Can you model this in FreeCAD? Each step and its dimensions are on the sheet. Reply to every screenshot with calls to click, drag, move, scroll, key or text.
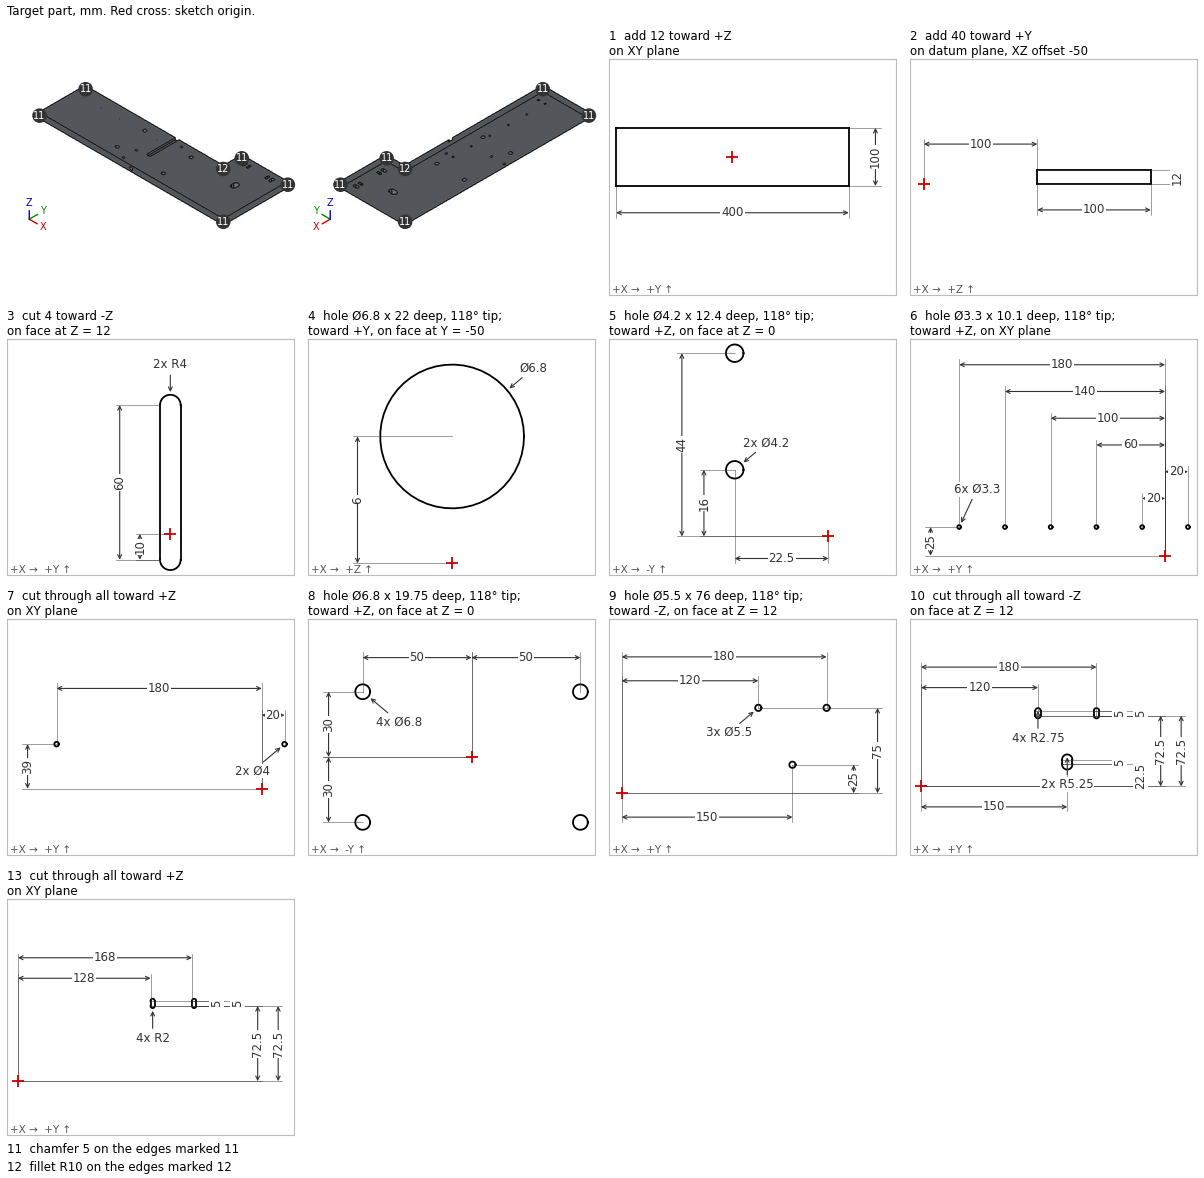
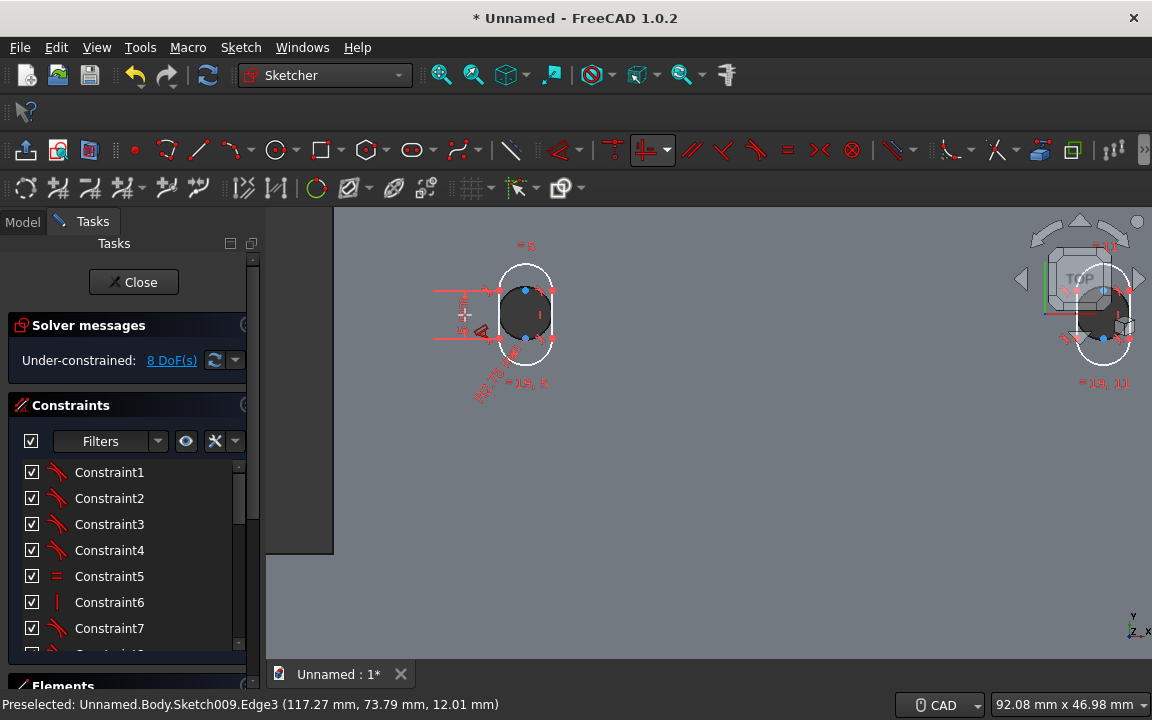
scroll(499, 325, down, 4)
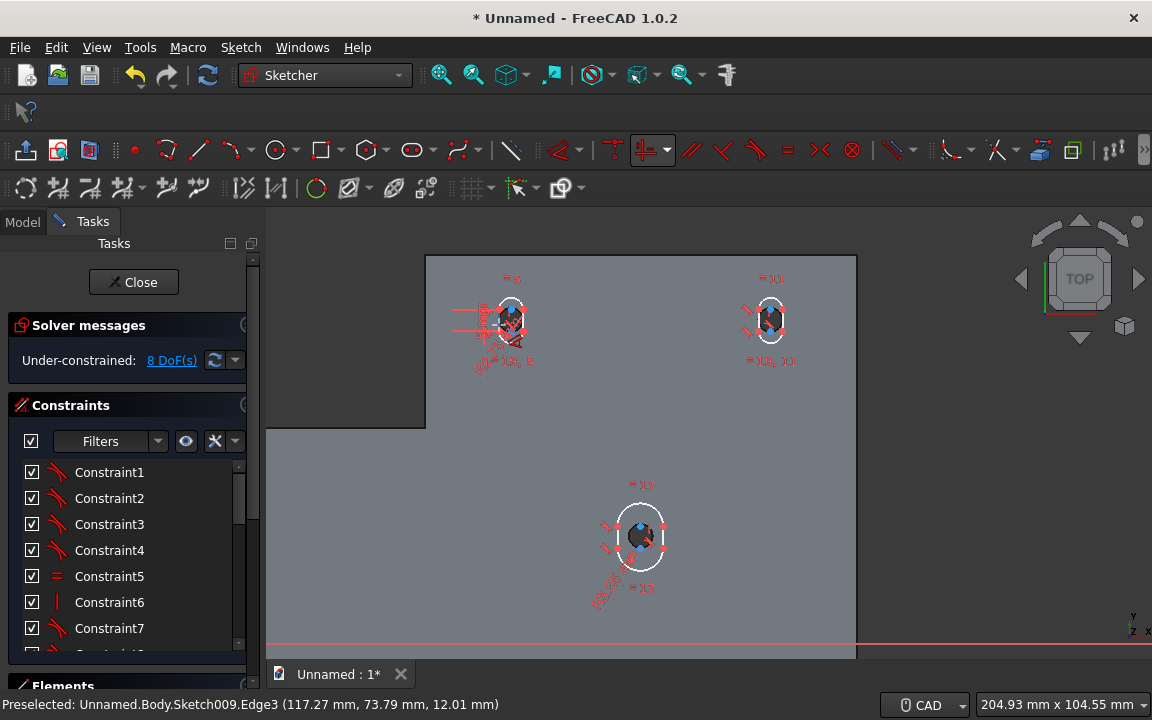
scroll(759, 325, up, 4)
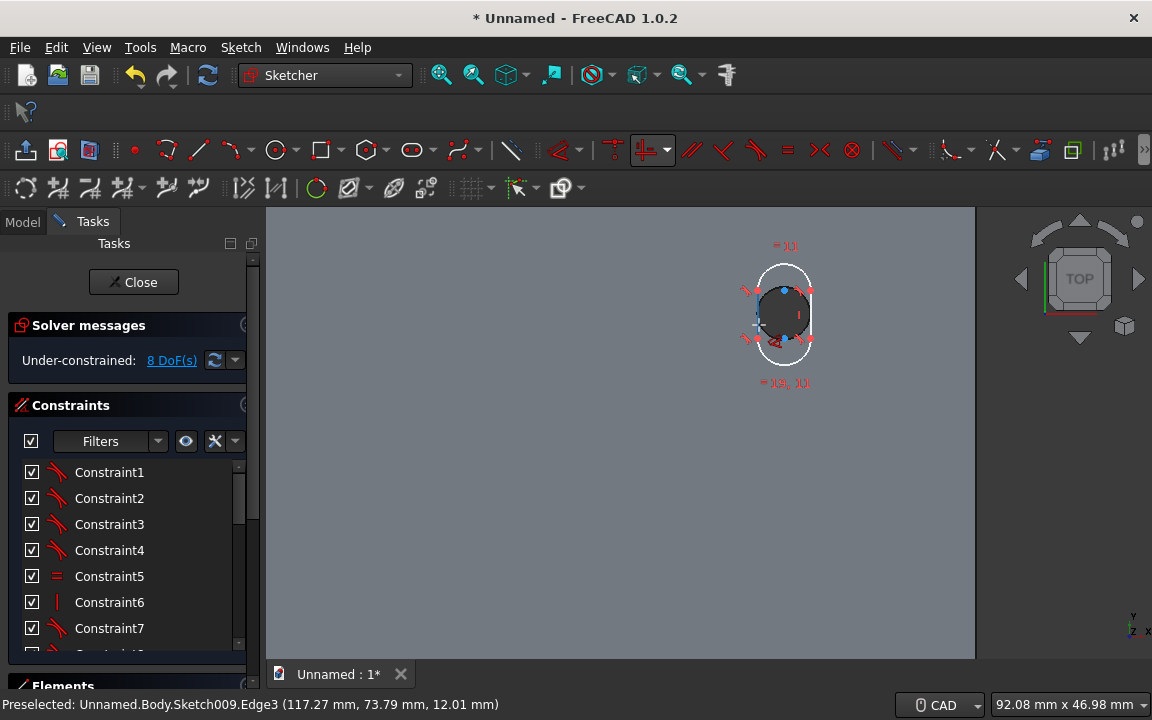
click(758, 324)
click(792, 315)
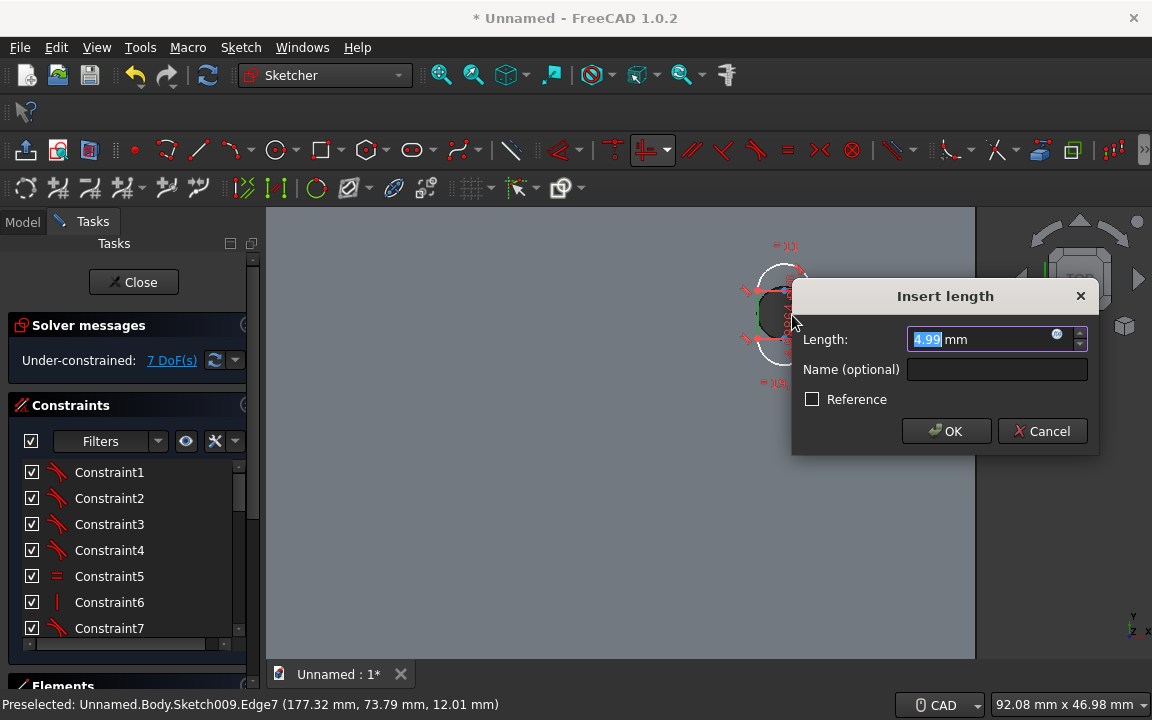
text(5)
key(Return)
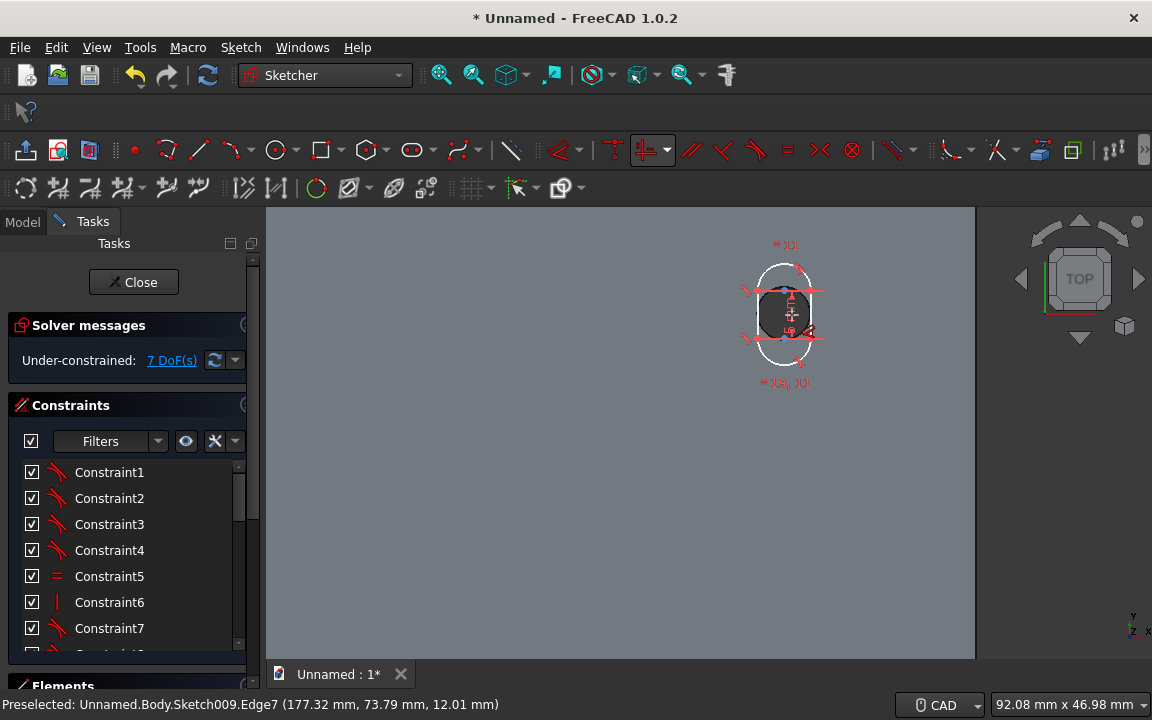
scroll(759, 325, down, 4)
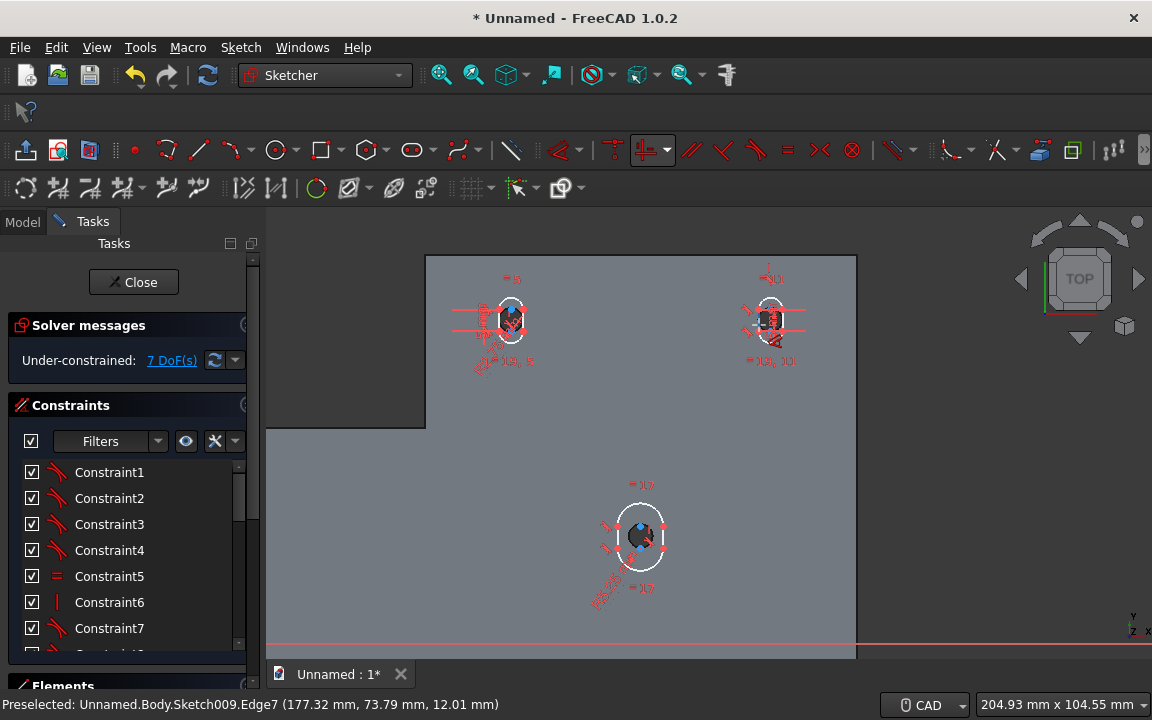
scroll(618, 542, up, 4)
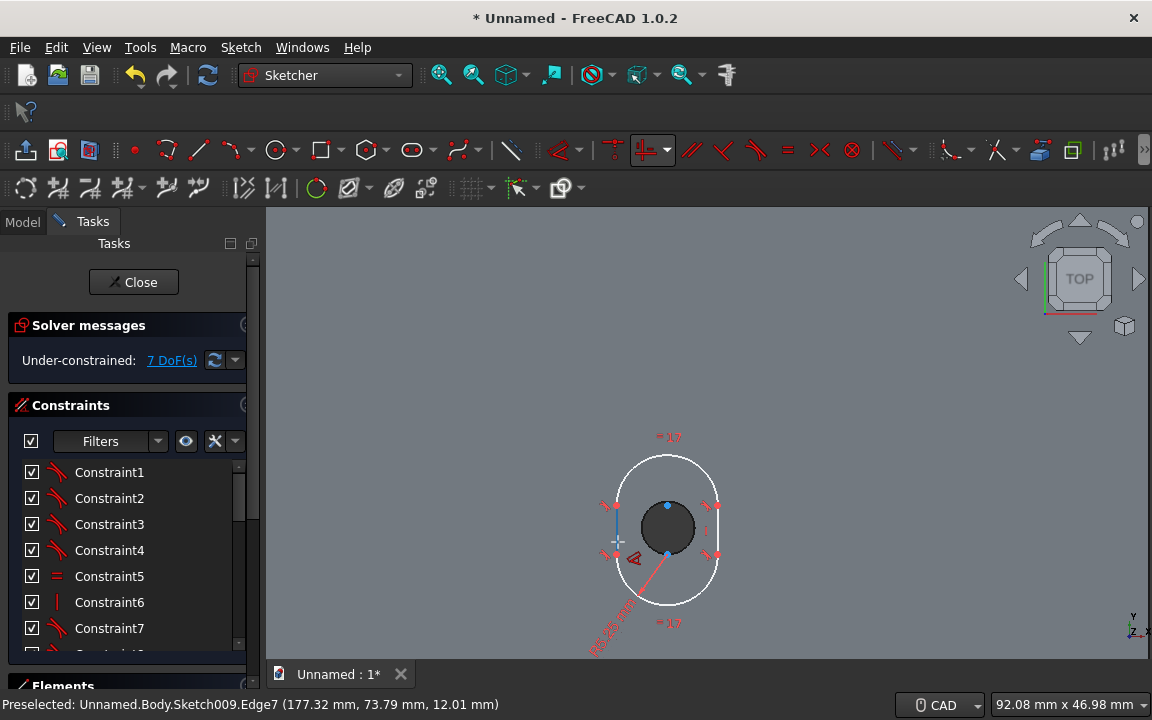
click(617, 540)
click(583, 530)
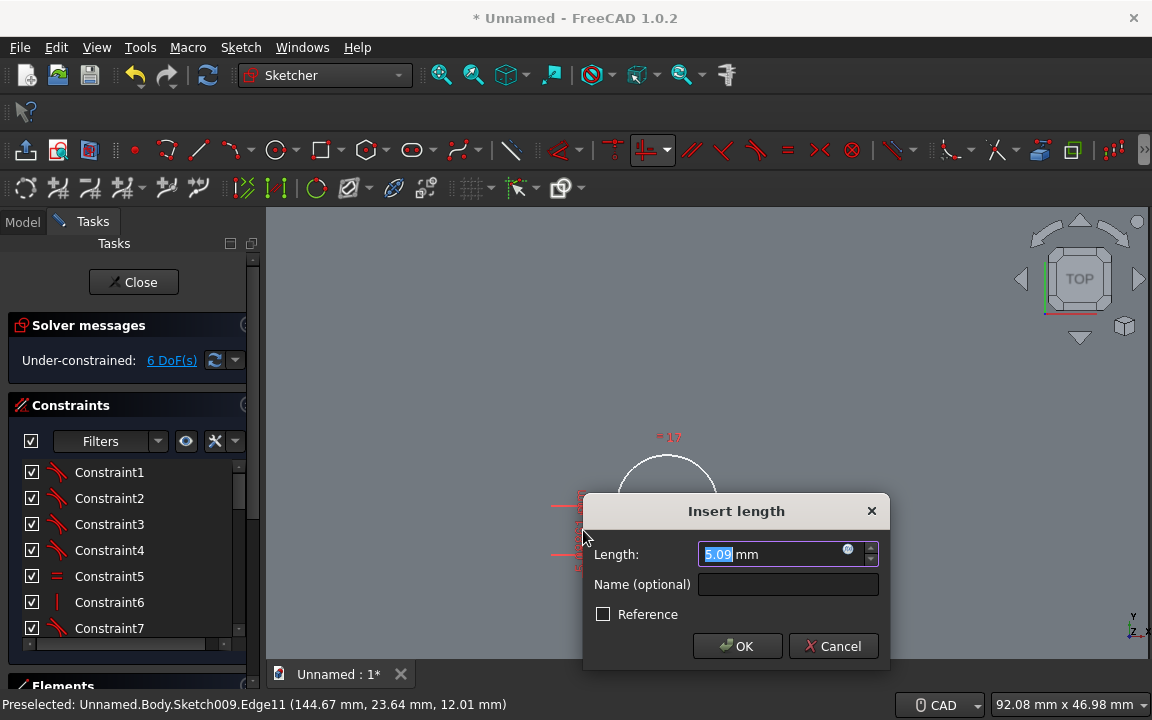
text(5)
key(Return)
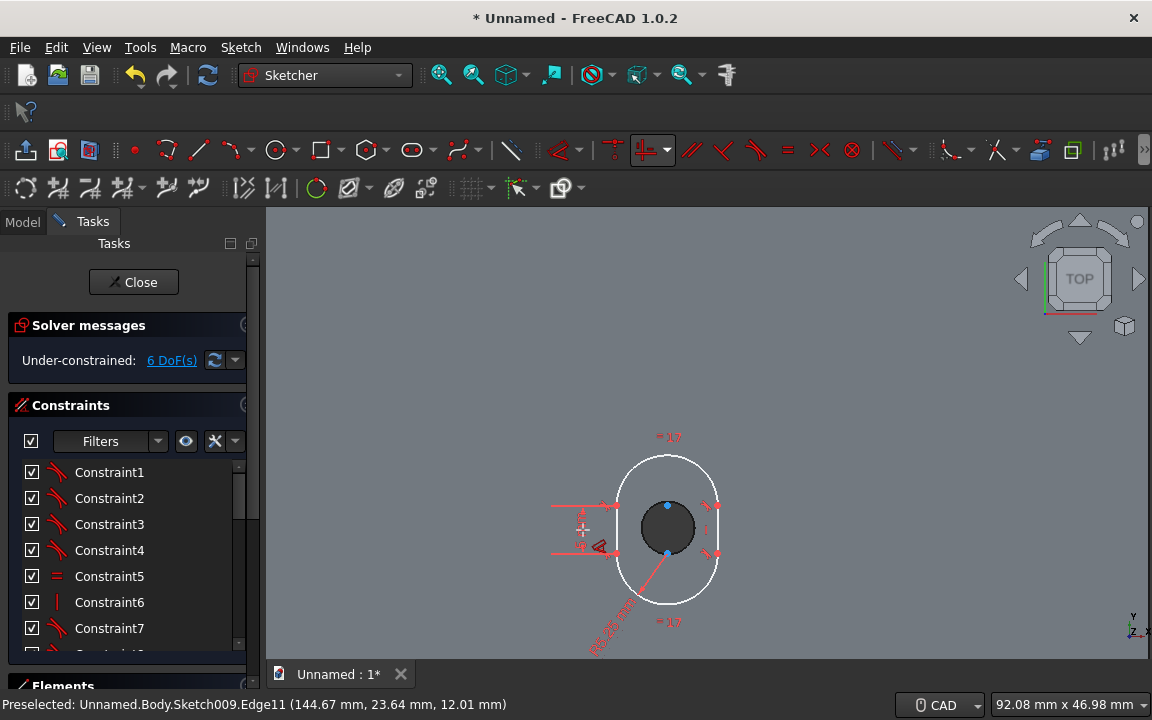
scroll(618, 542, down, 4)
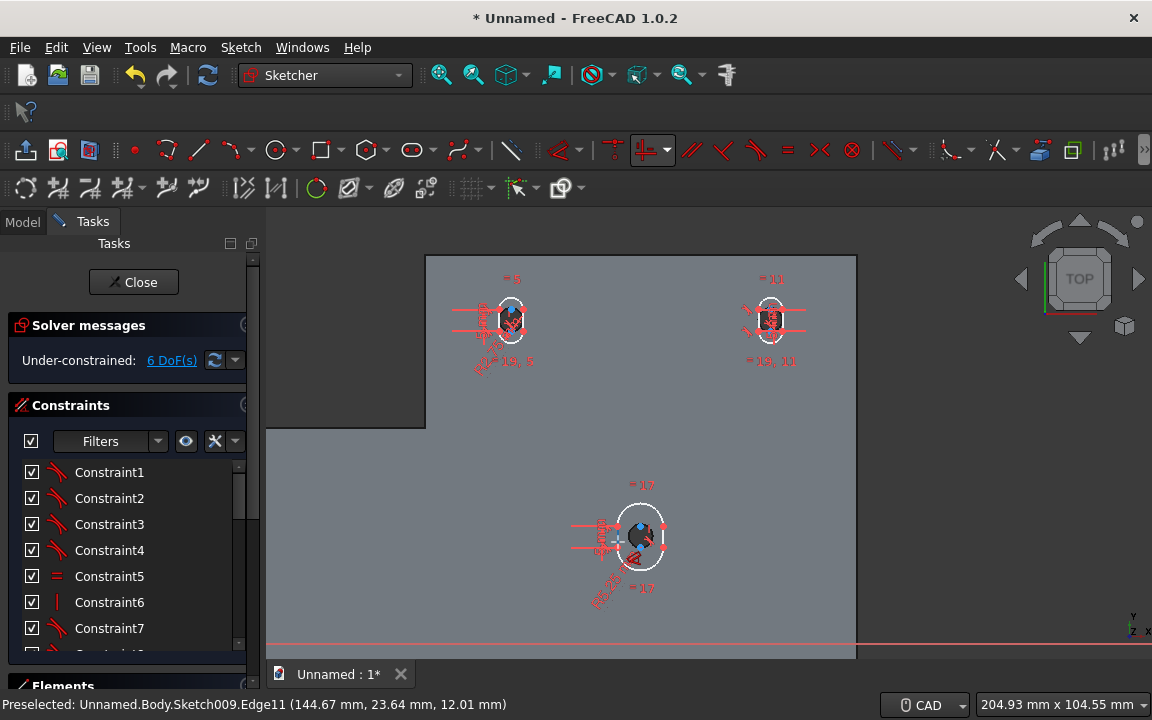
click(511, 331)
click(403, 297)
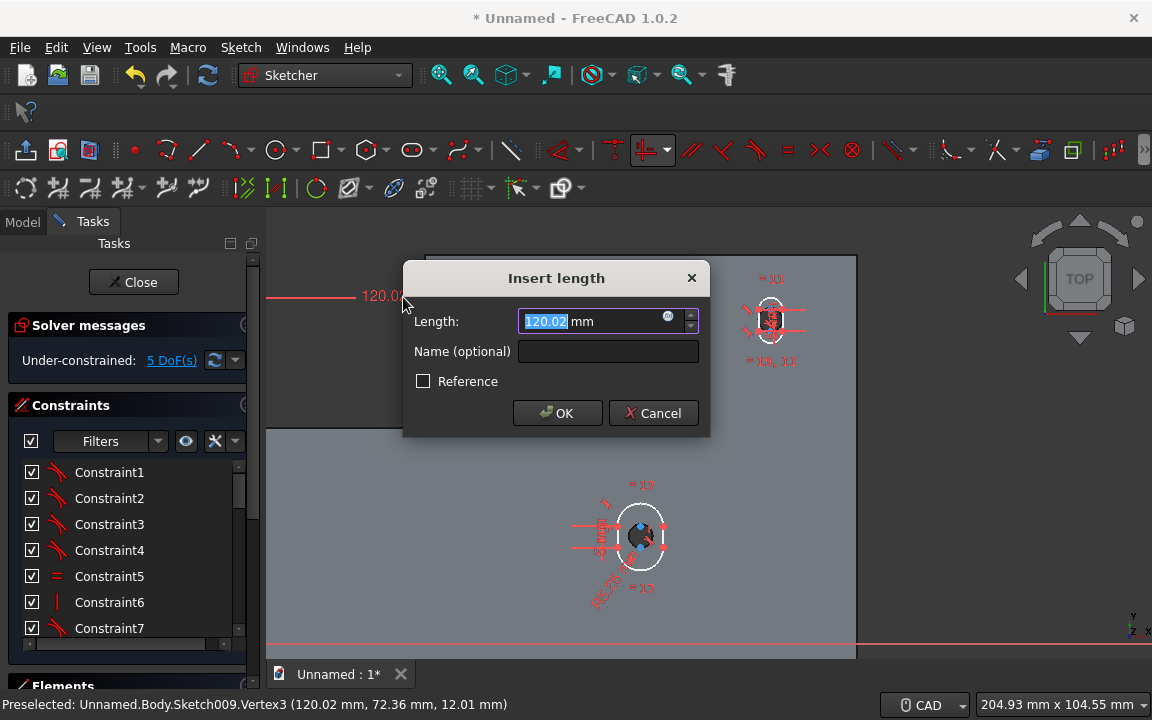
text(120)
key(Return)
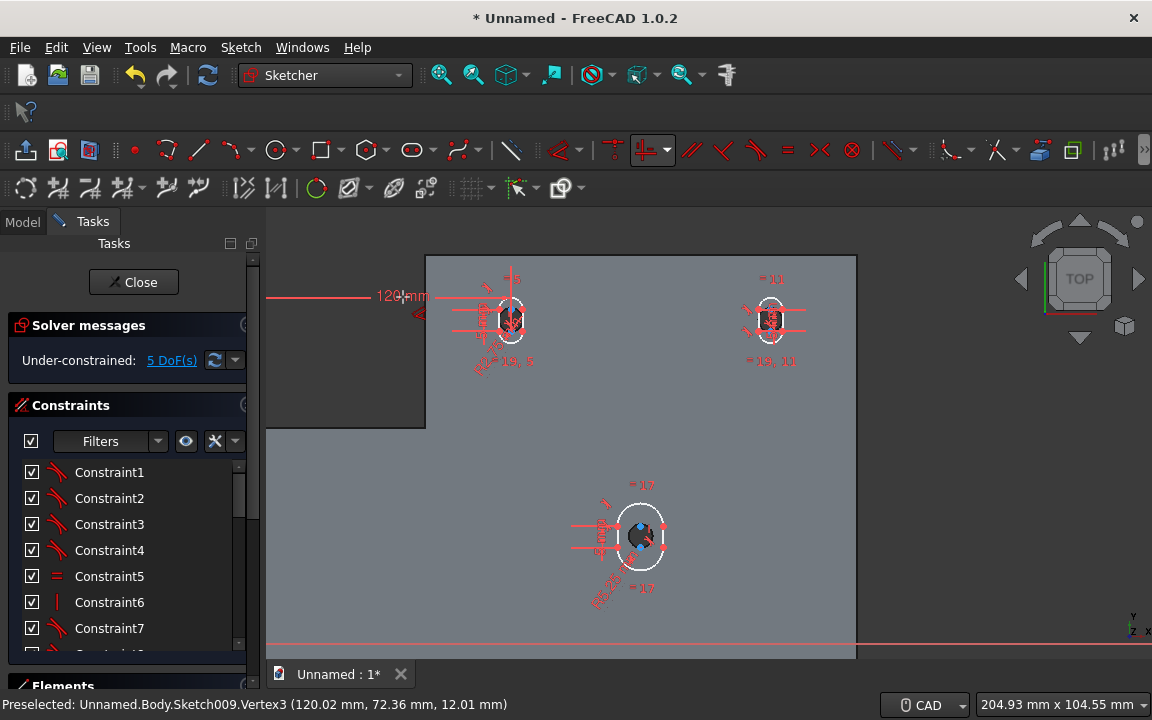
click(771, 331)
click(642, 297)